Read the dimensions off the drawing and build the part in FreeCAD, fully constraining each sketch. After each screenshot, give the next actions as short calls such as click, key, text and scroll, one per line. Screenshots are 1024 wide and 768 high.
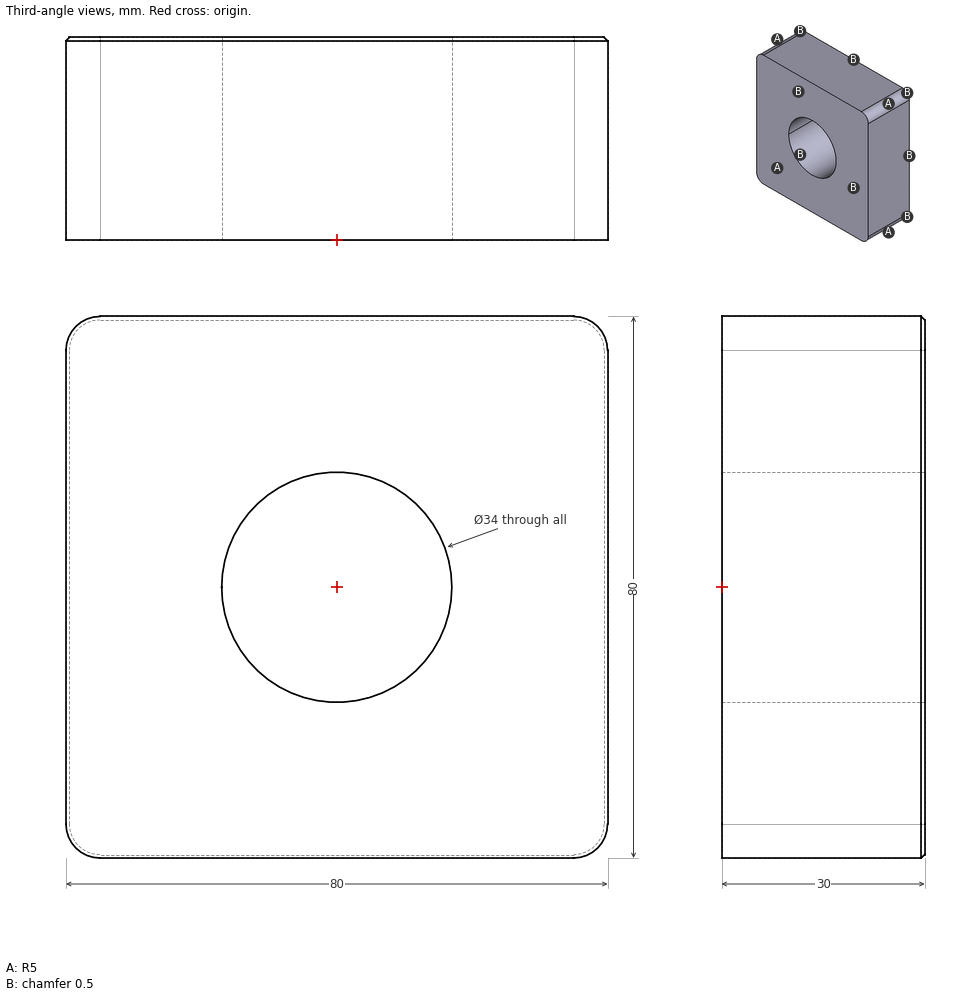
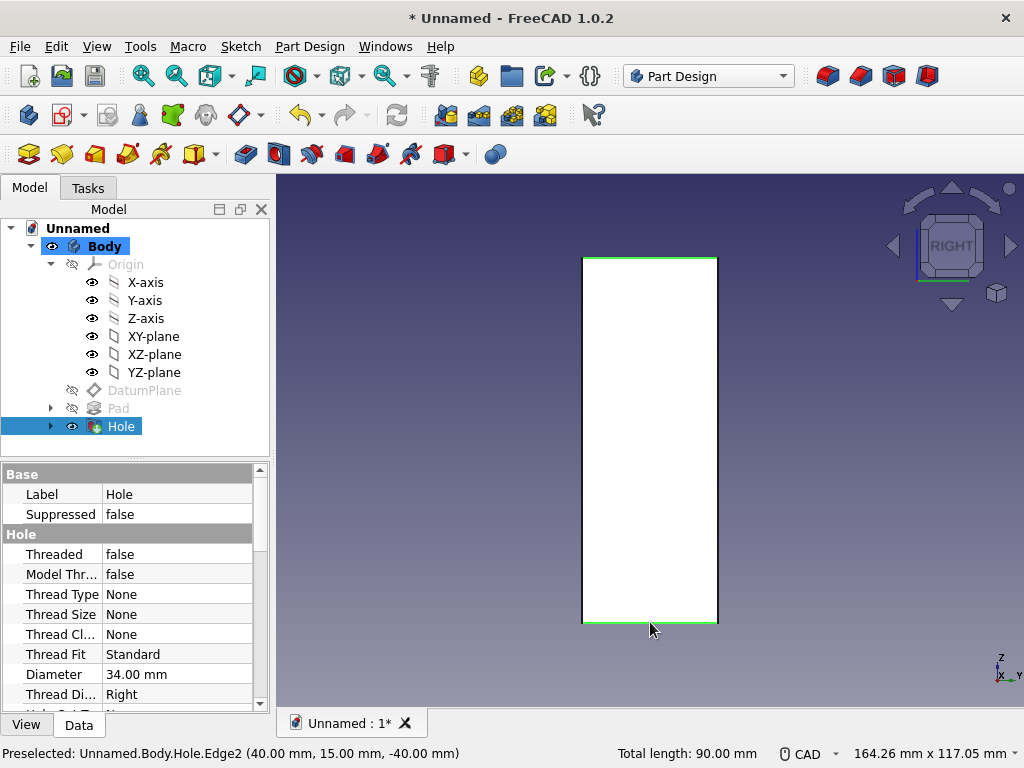
key(5)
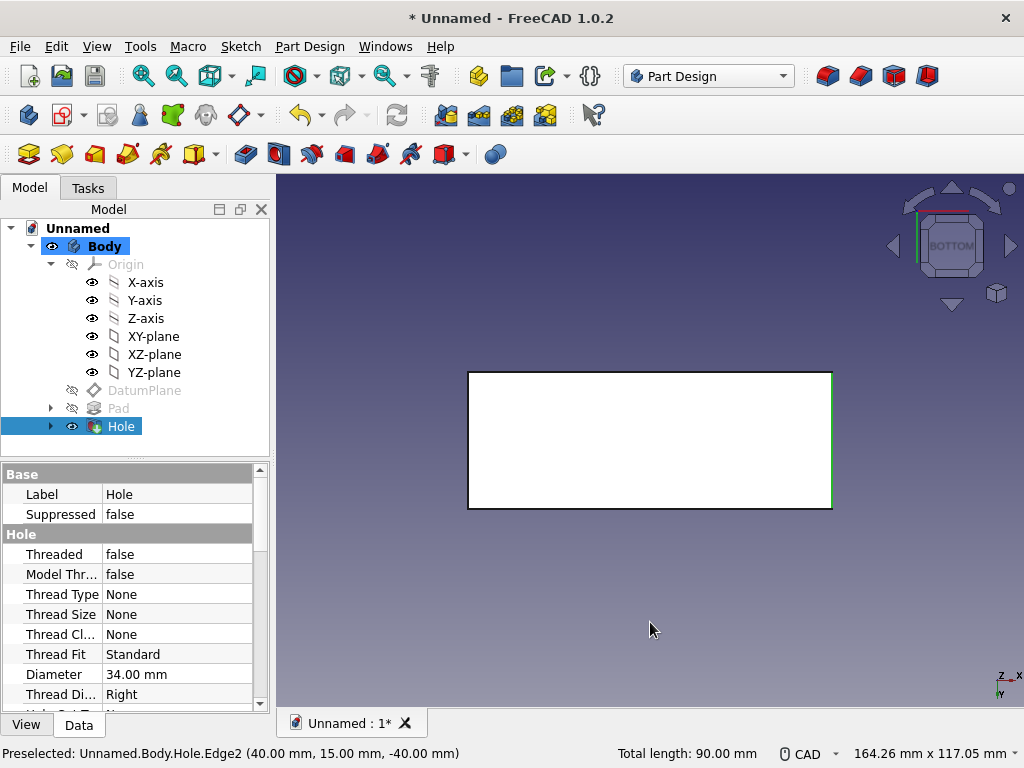
click(468, 440, ctrl)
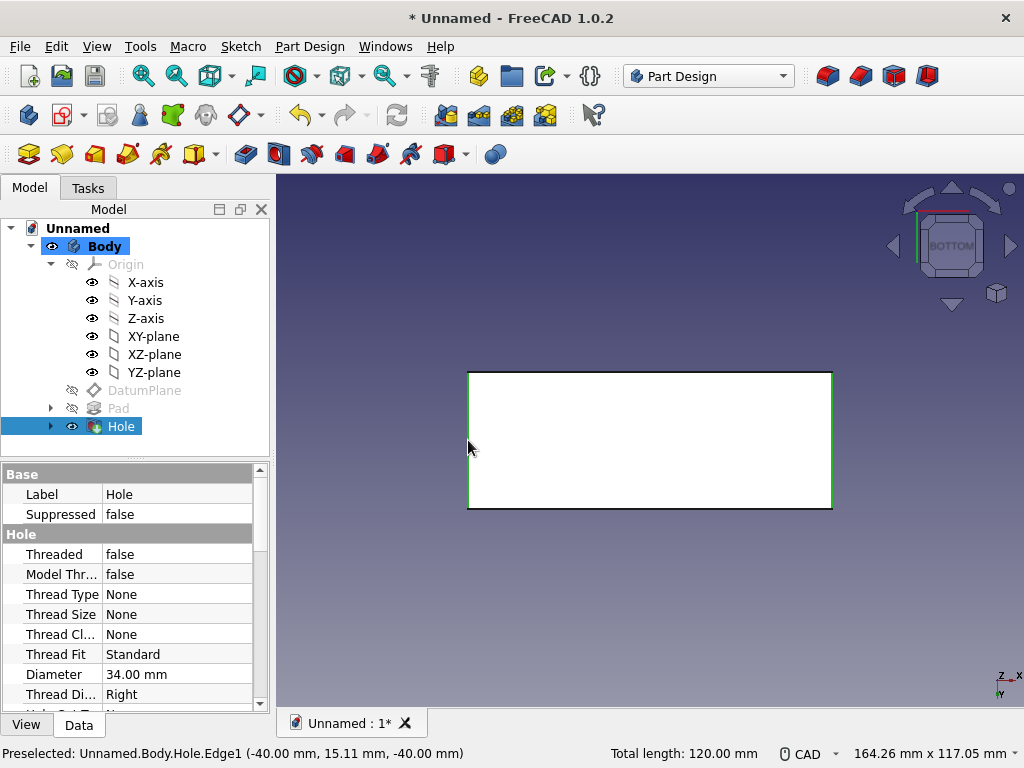
click(828, 76)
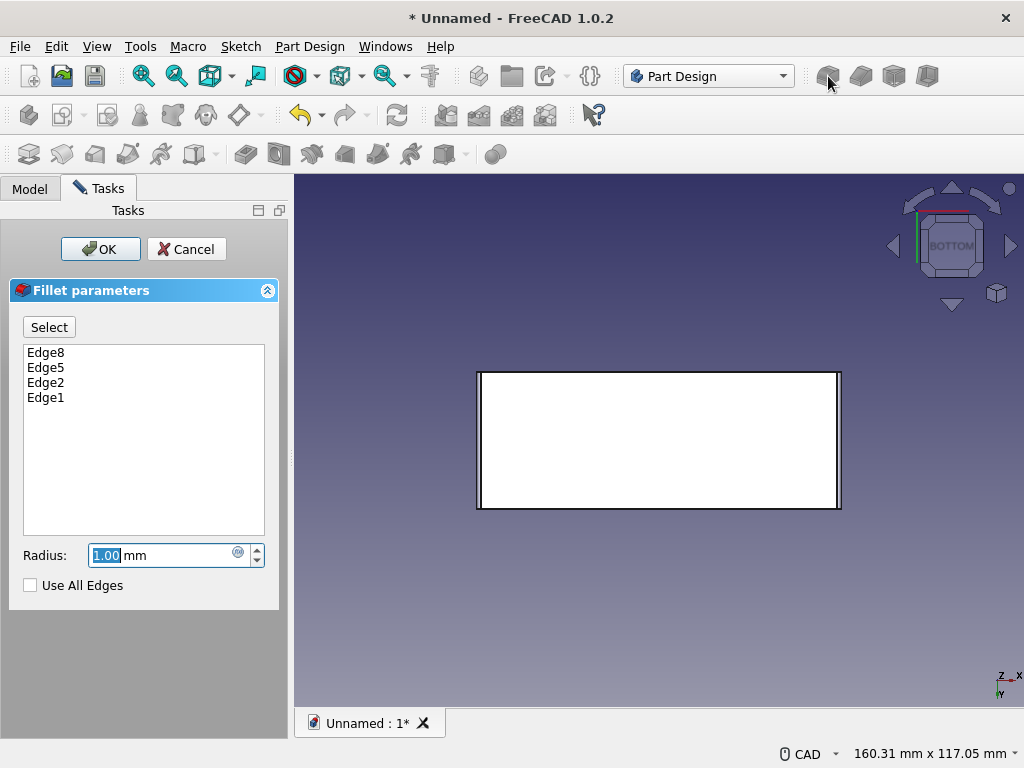
text(5)
key(Tab)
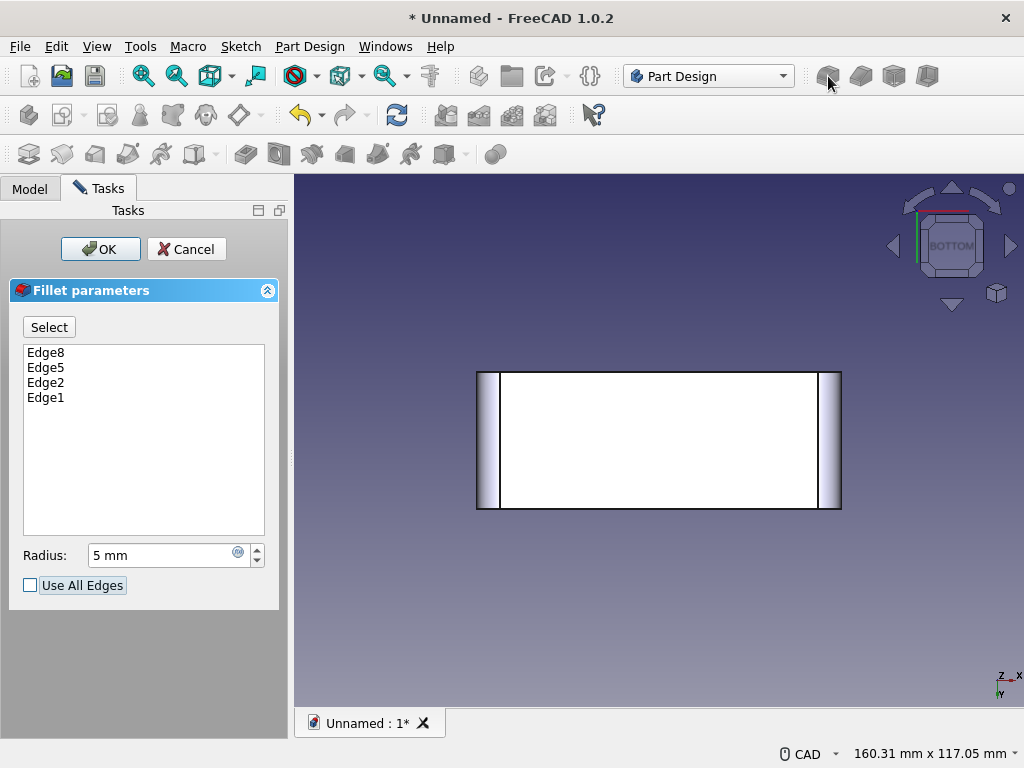
click(101, 249)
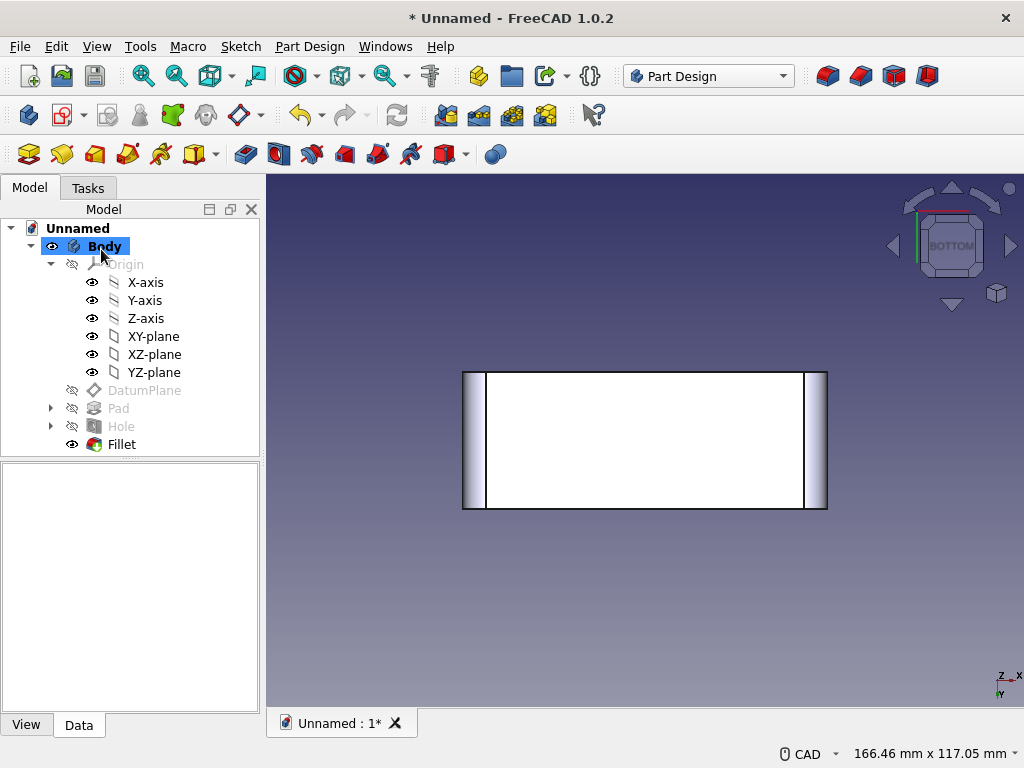
click(470, 508)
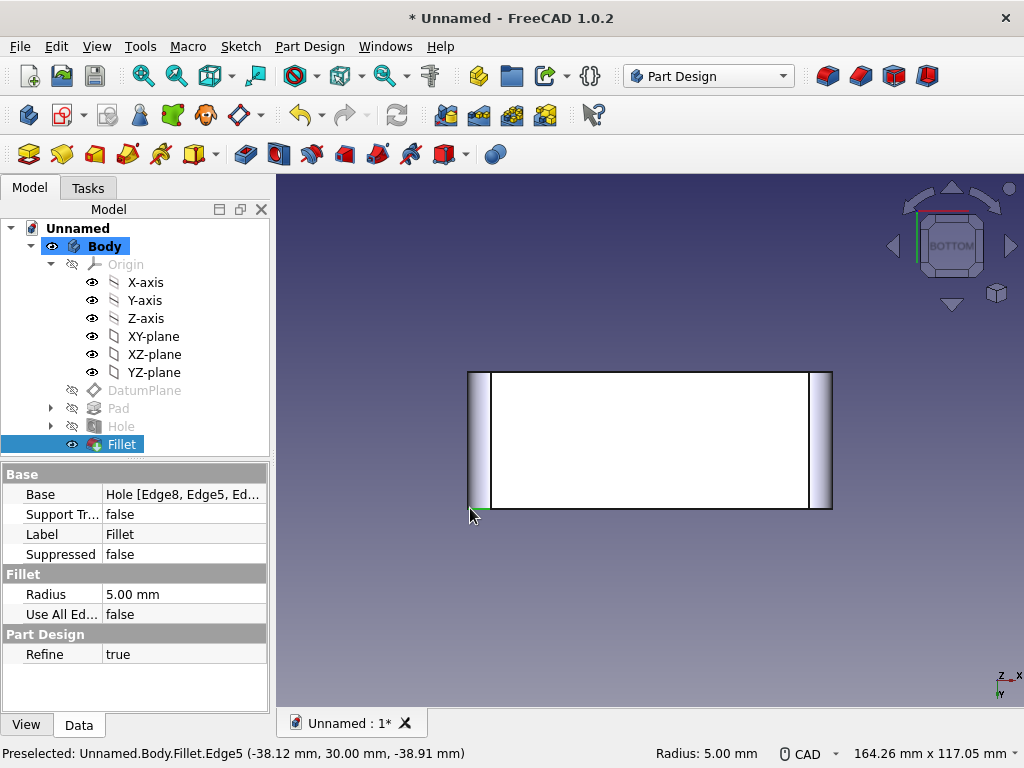
click(825, 508, ctrl)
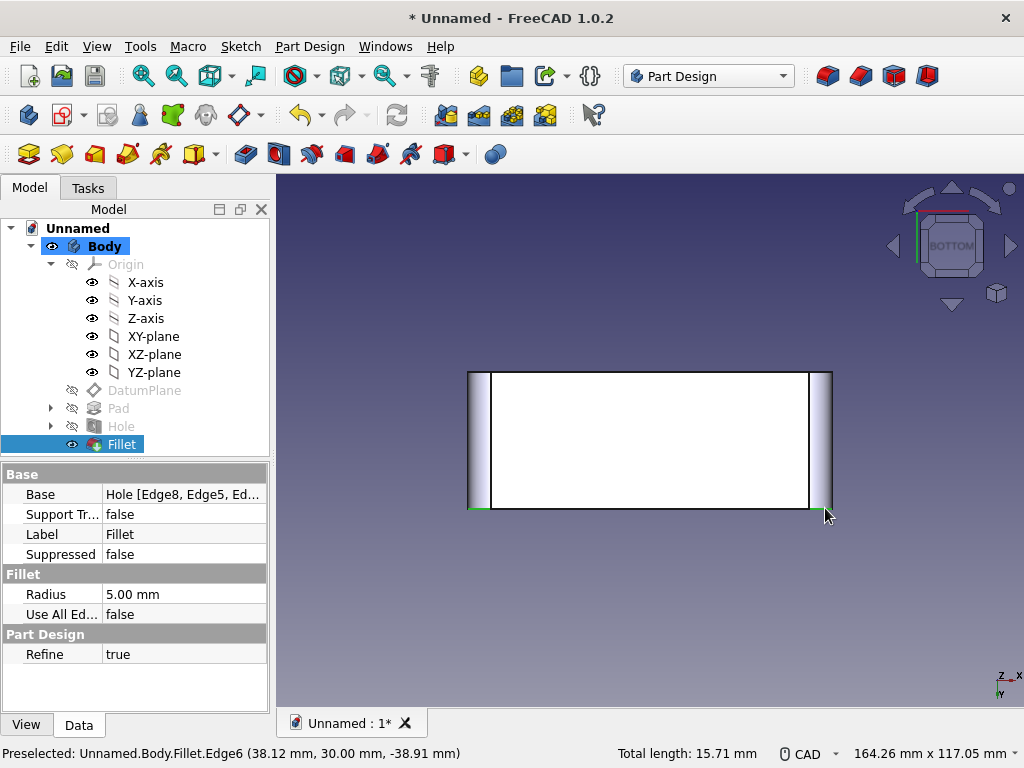
key(0)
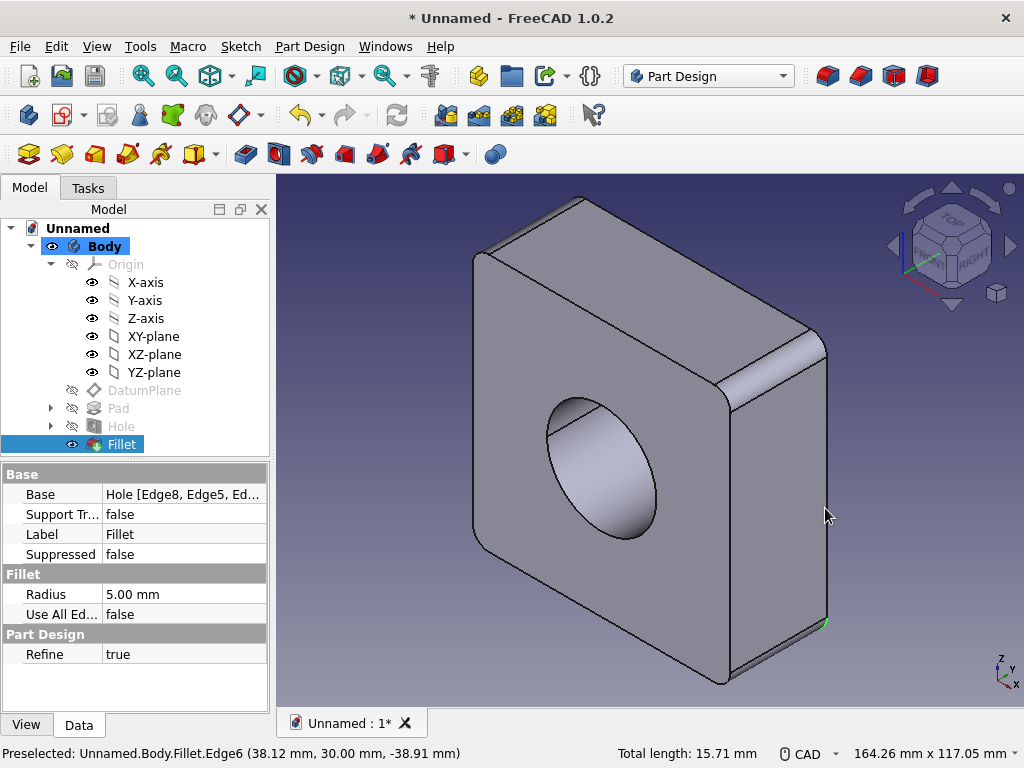
key(2)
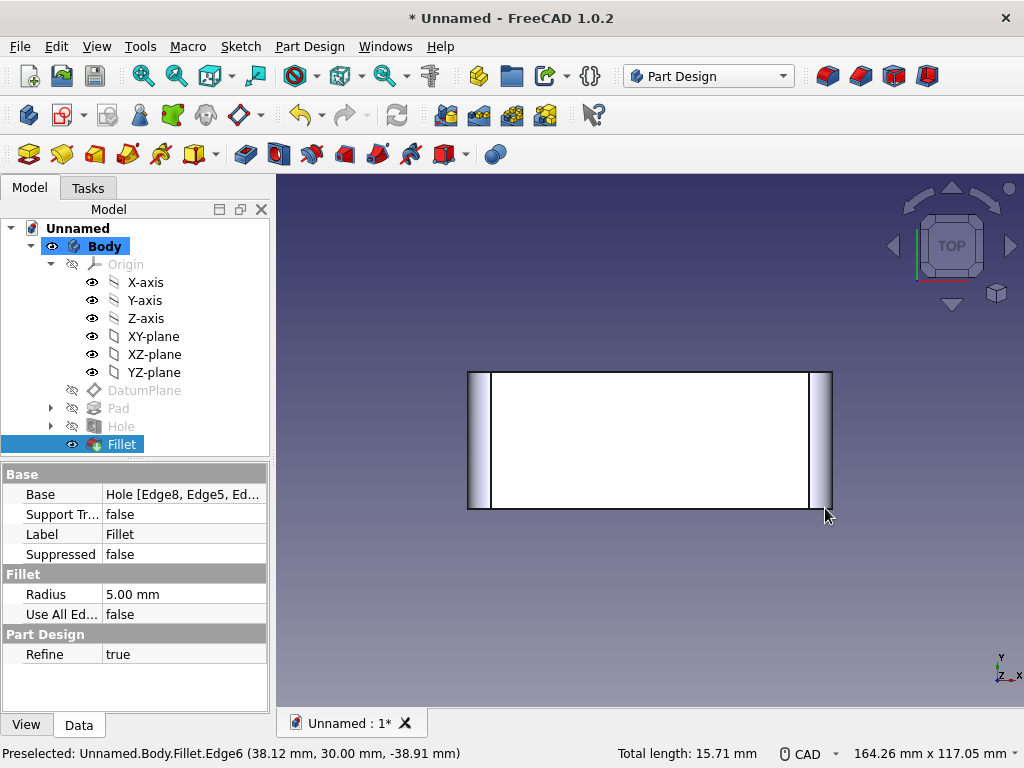
click(650, 371, ctrl)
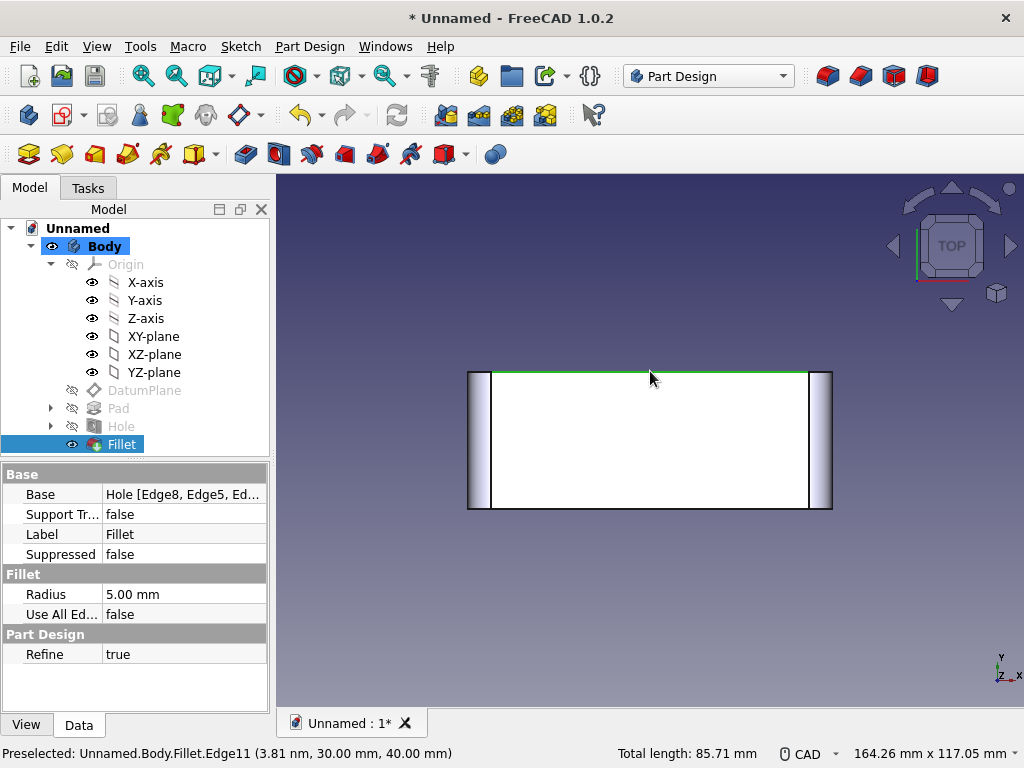
click(475, 371, ctrl)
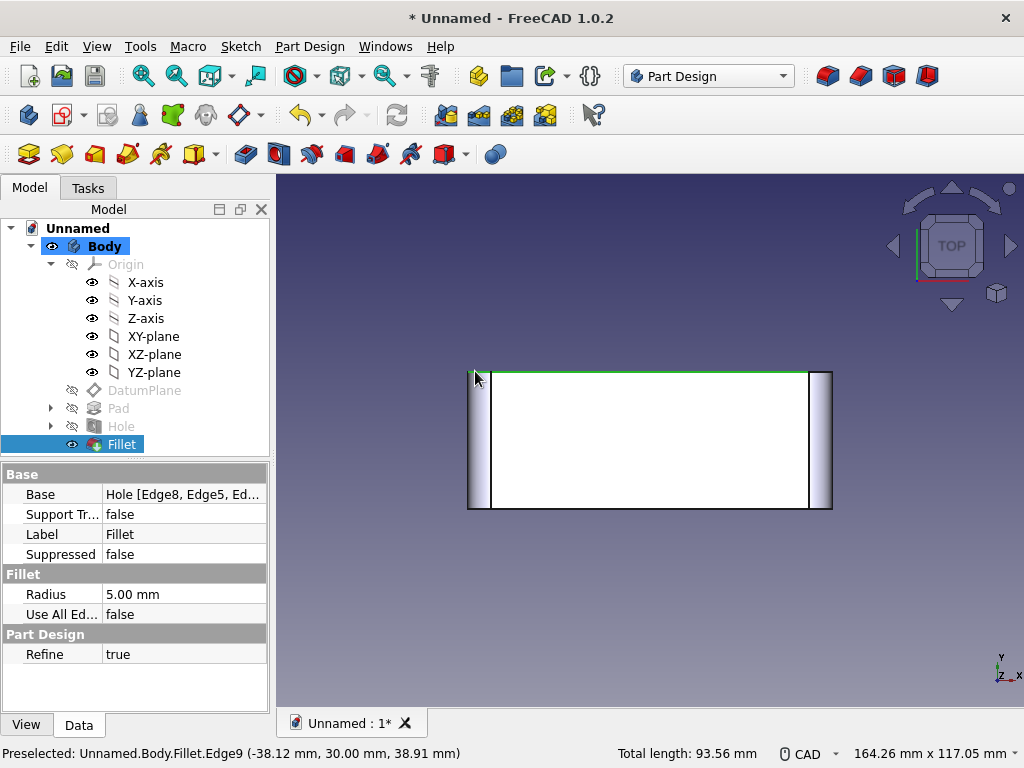
click(825, 371, ctrl)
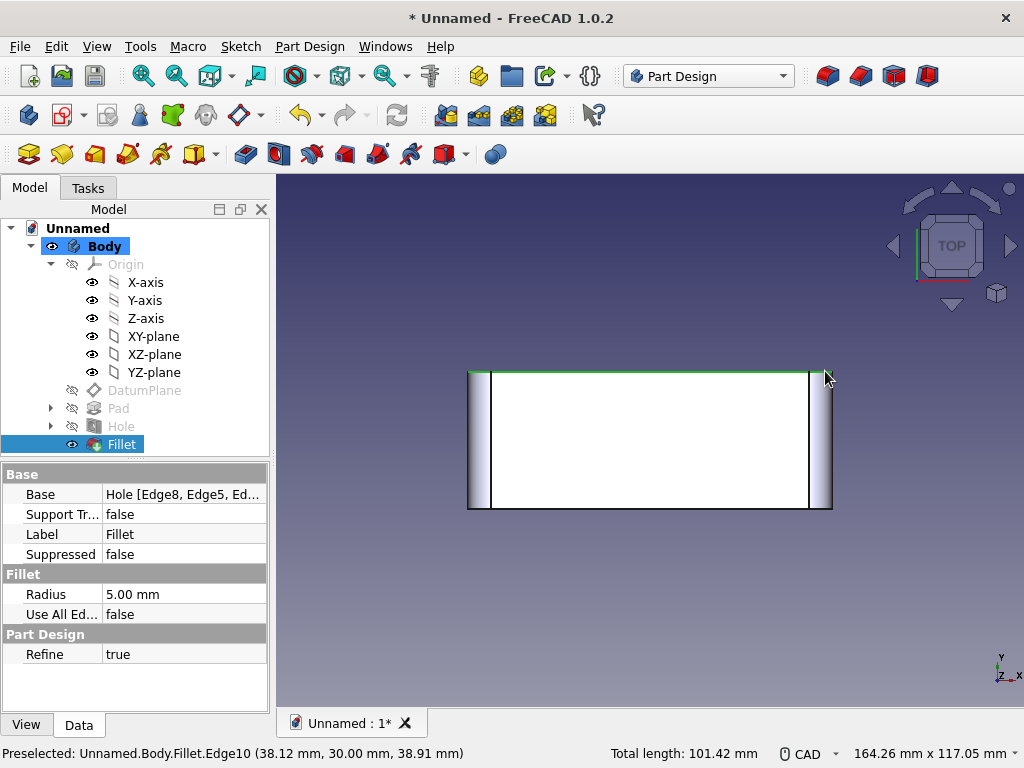
key(1)